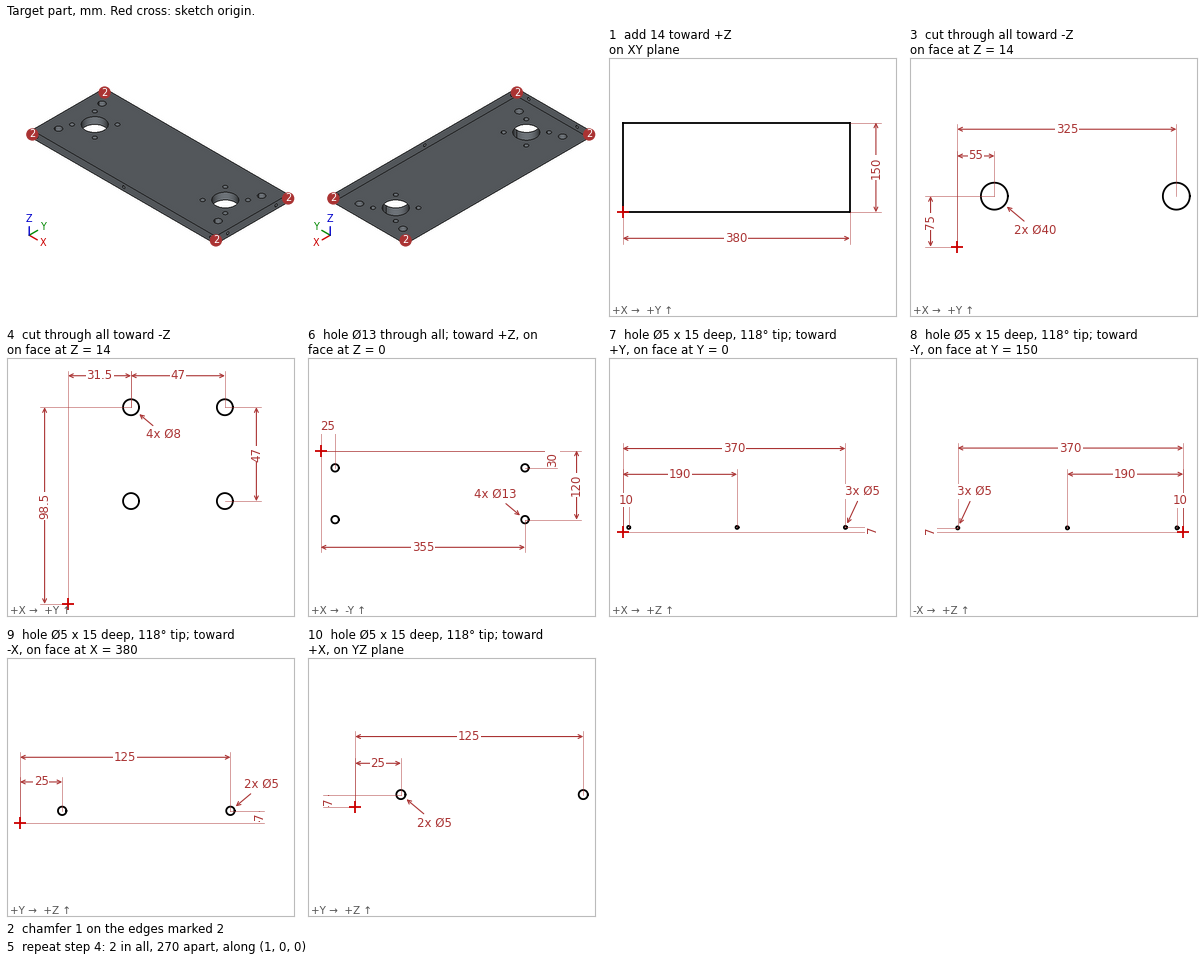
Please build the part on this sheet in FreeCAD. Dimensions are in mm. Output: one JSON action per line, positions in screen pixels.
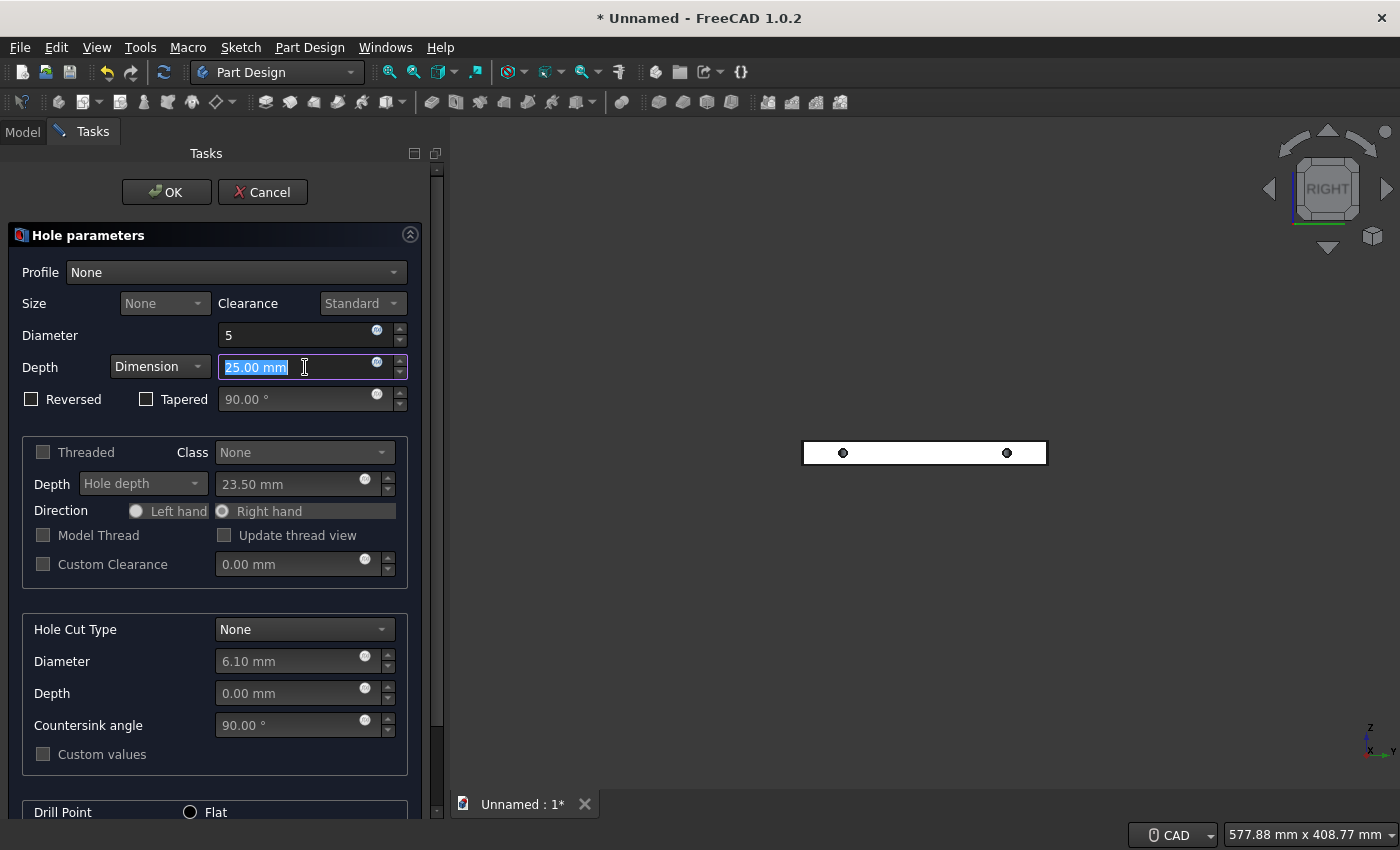
{"action": "type", "text": "15"}
{"action": "key", "text": "Tab"}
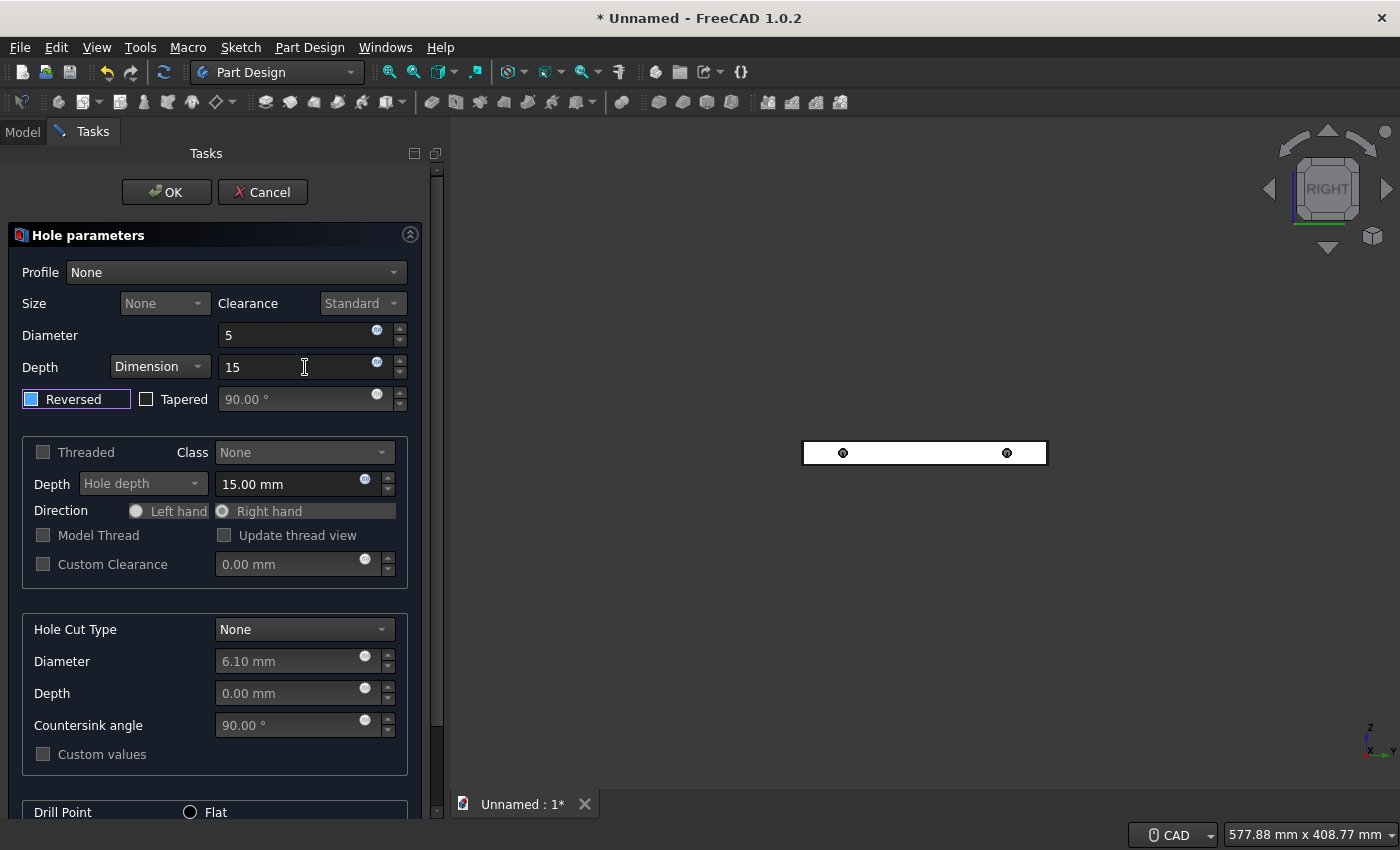
{"action": "left_click", "coordinate": [167, 192]}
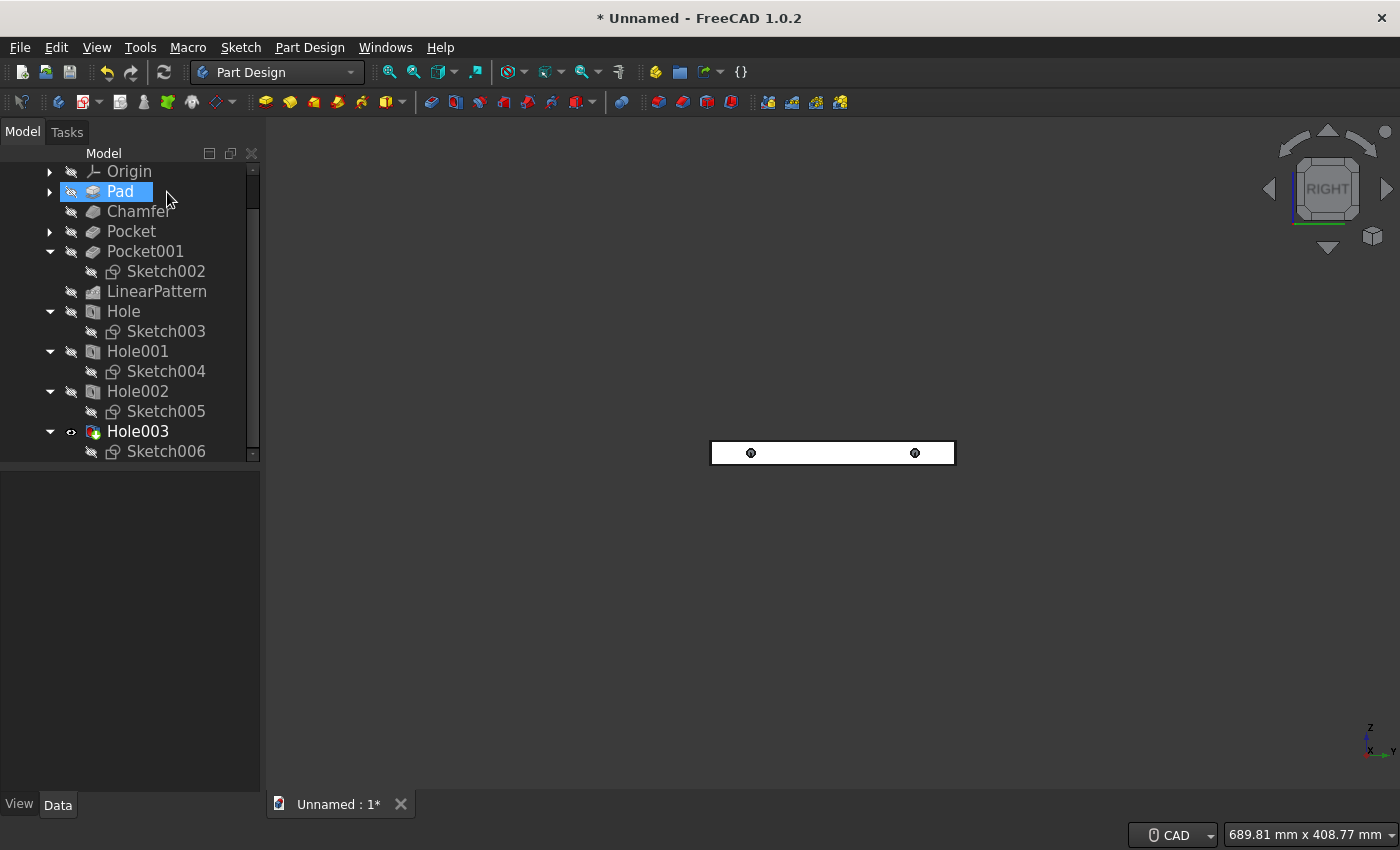
{"action": "key", "text": "v f"}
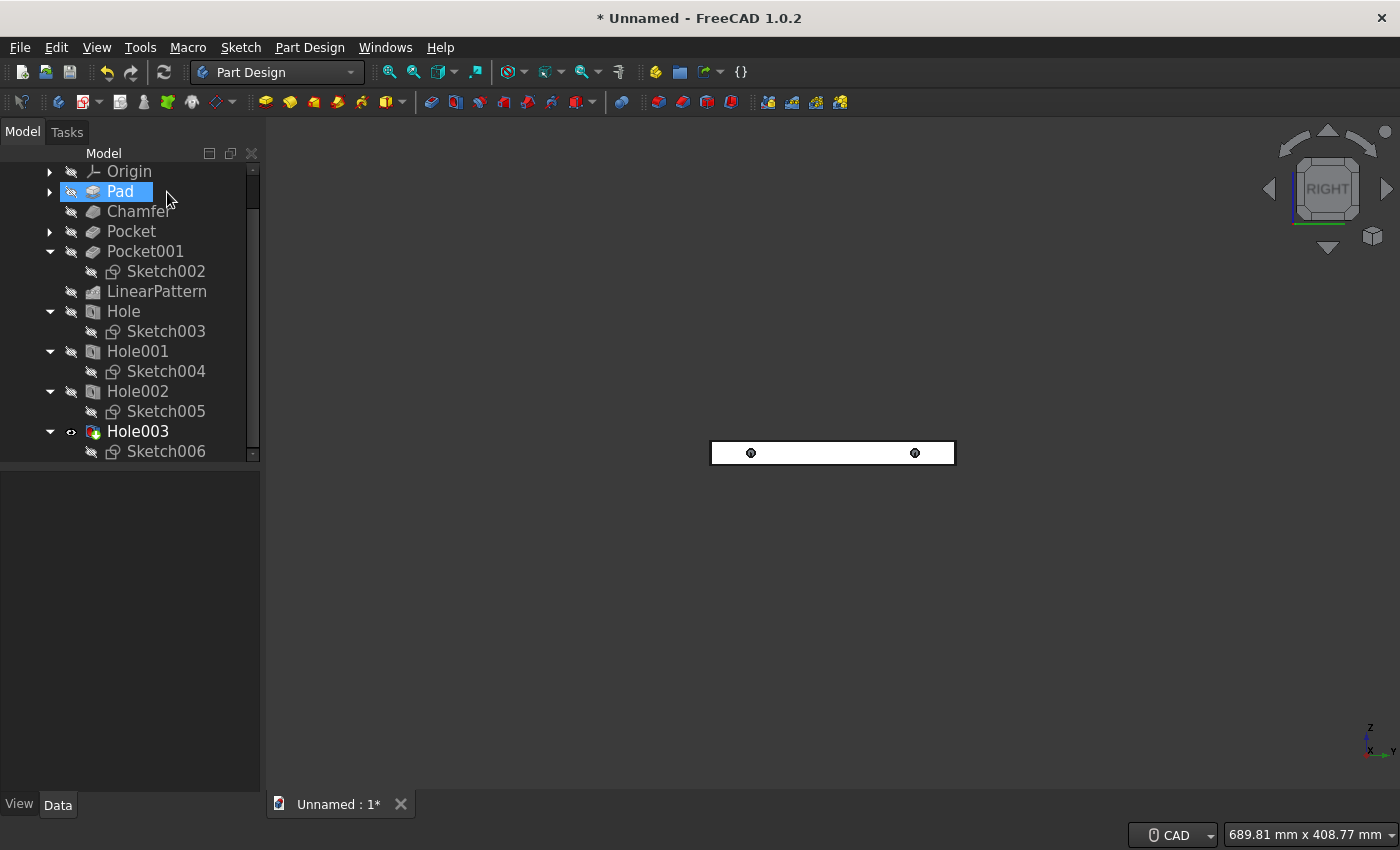
{"action": "left_click", "coordinate": [84, 102]}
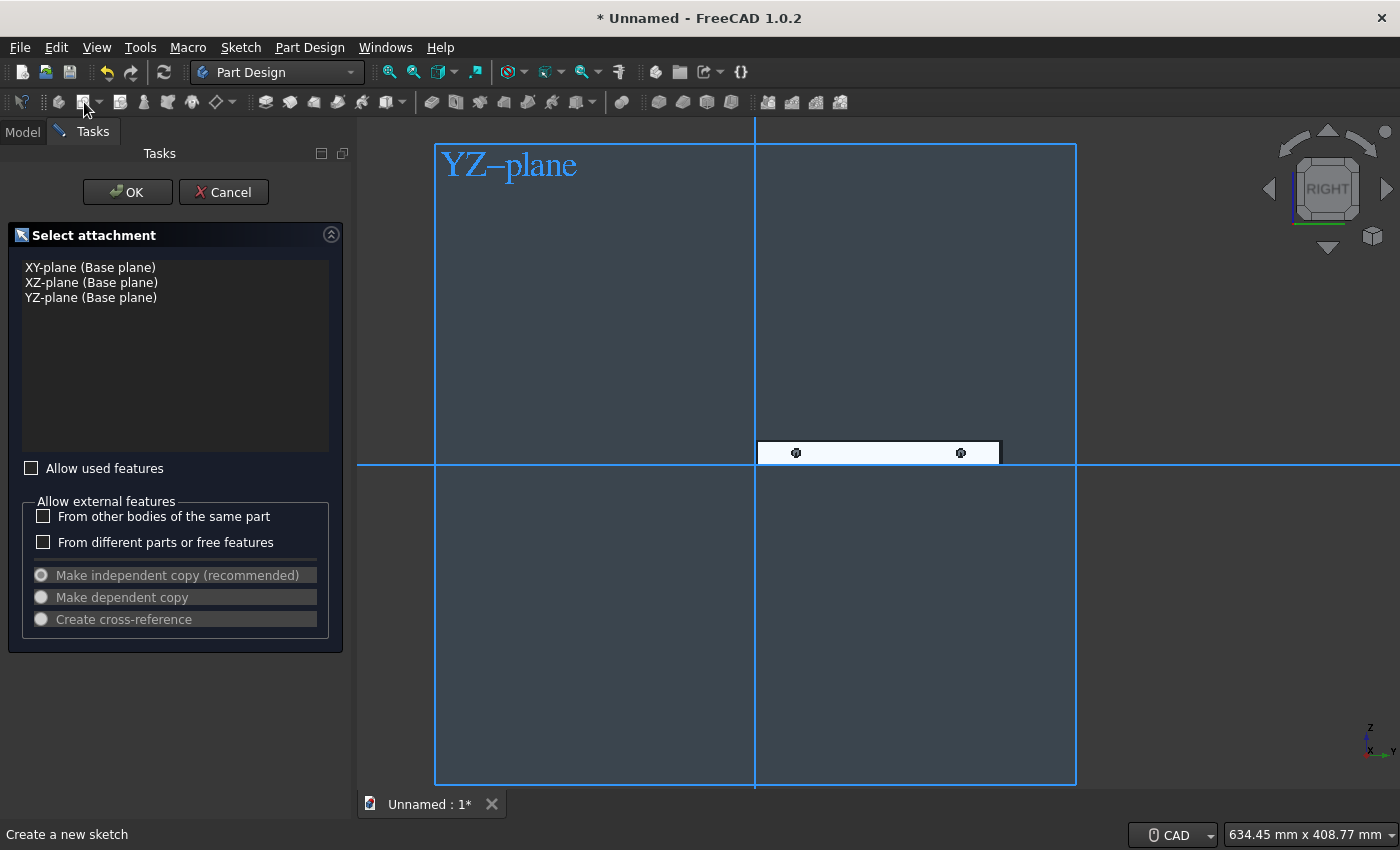
{"action": "left_click", "coordinate": [82, 298]}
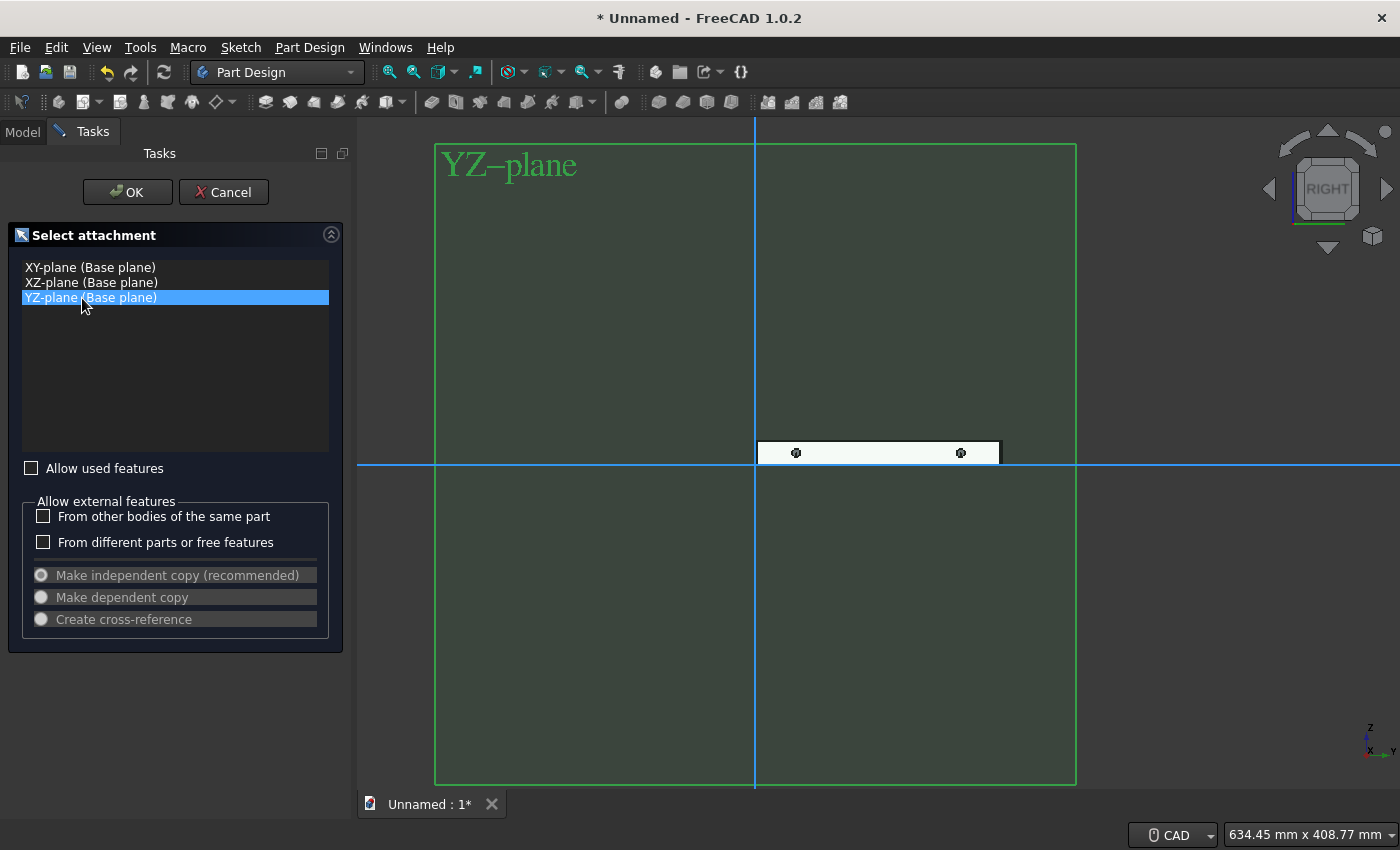
{"action": "left_click", "coordinate": [128, 192]}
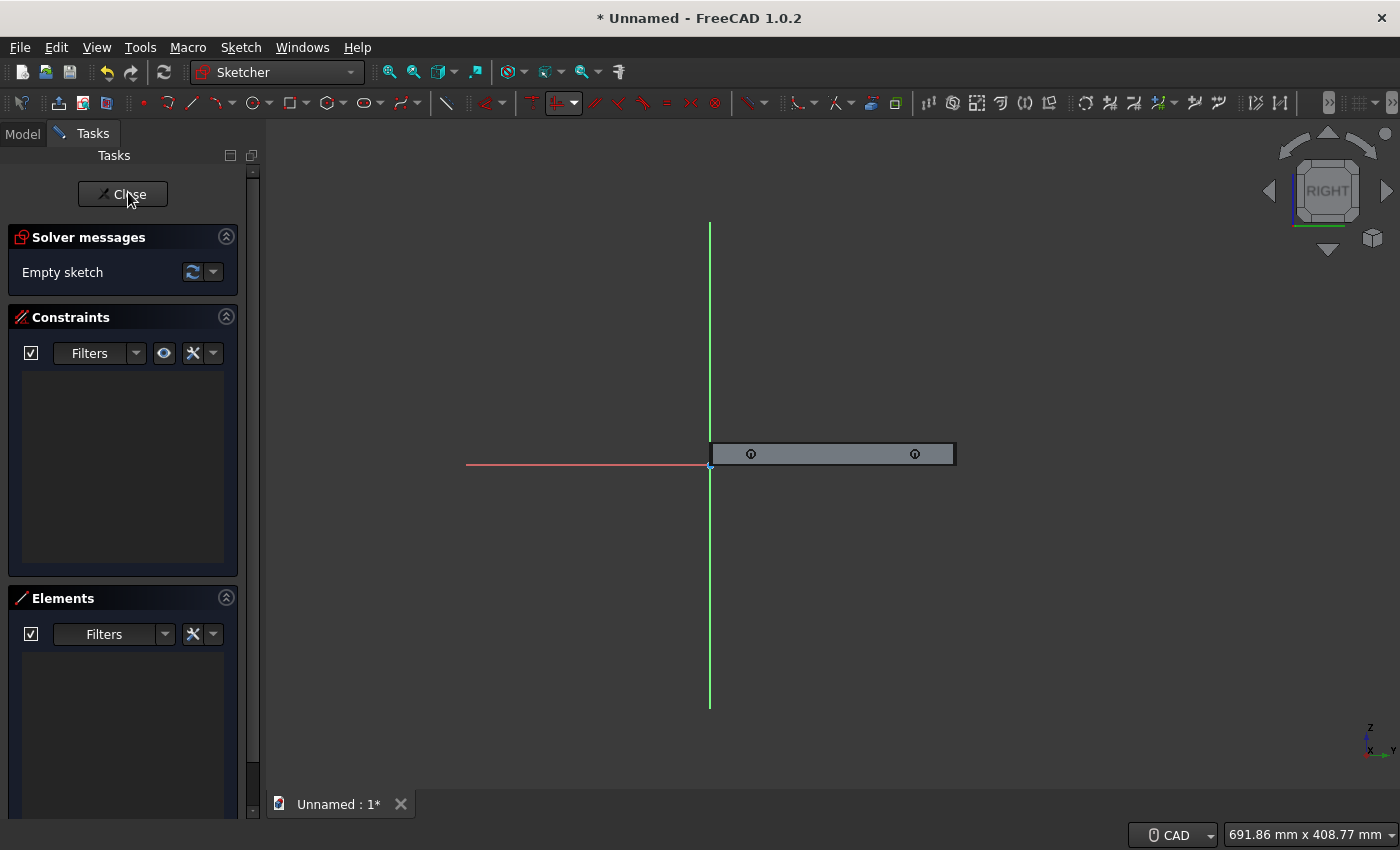
{"action": "key", "text": "q s"}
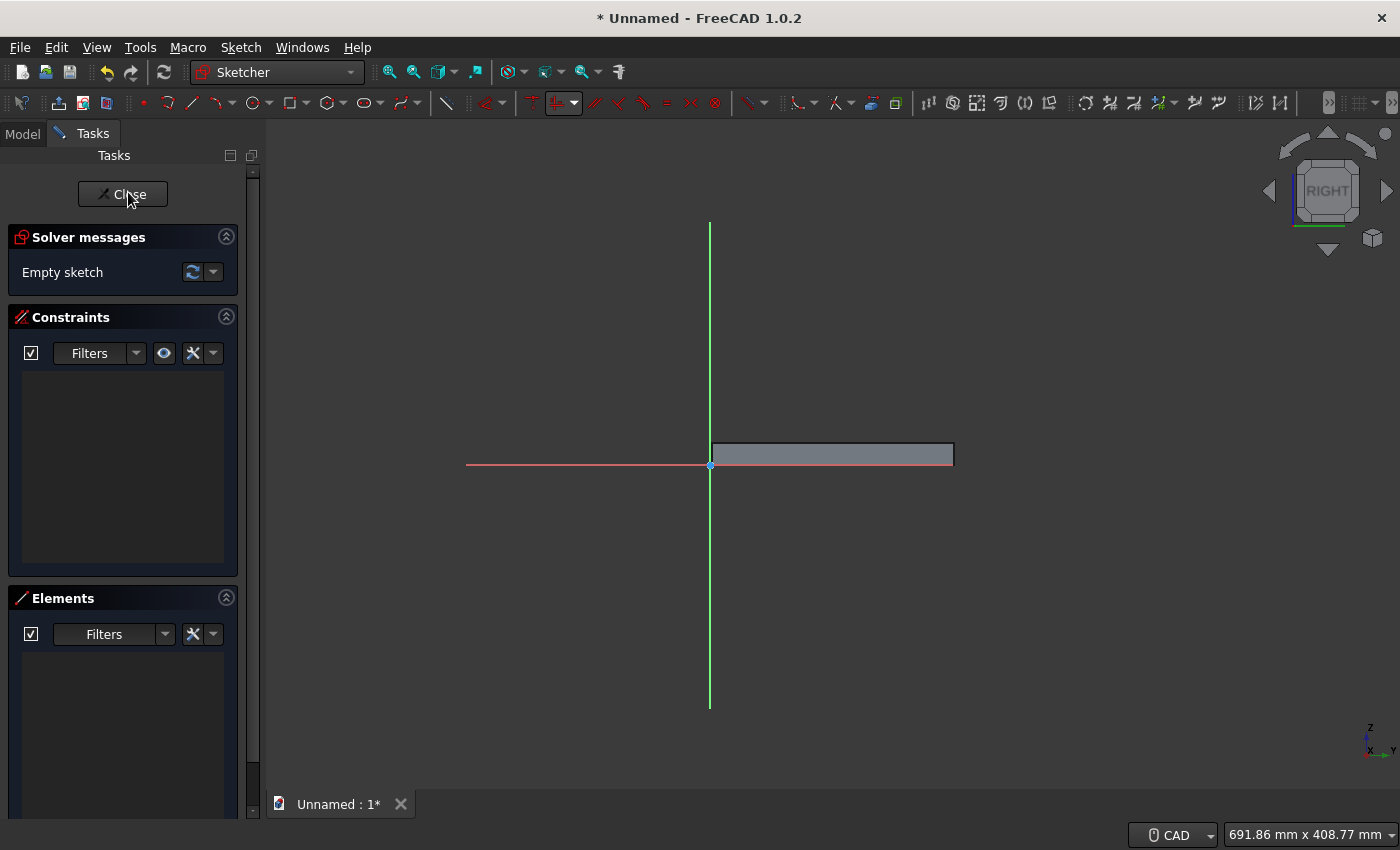
{"action": "scroll", "coordinate": [836, 459], "scroll_direction": "up", "scroll_amount": 6}